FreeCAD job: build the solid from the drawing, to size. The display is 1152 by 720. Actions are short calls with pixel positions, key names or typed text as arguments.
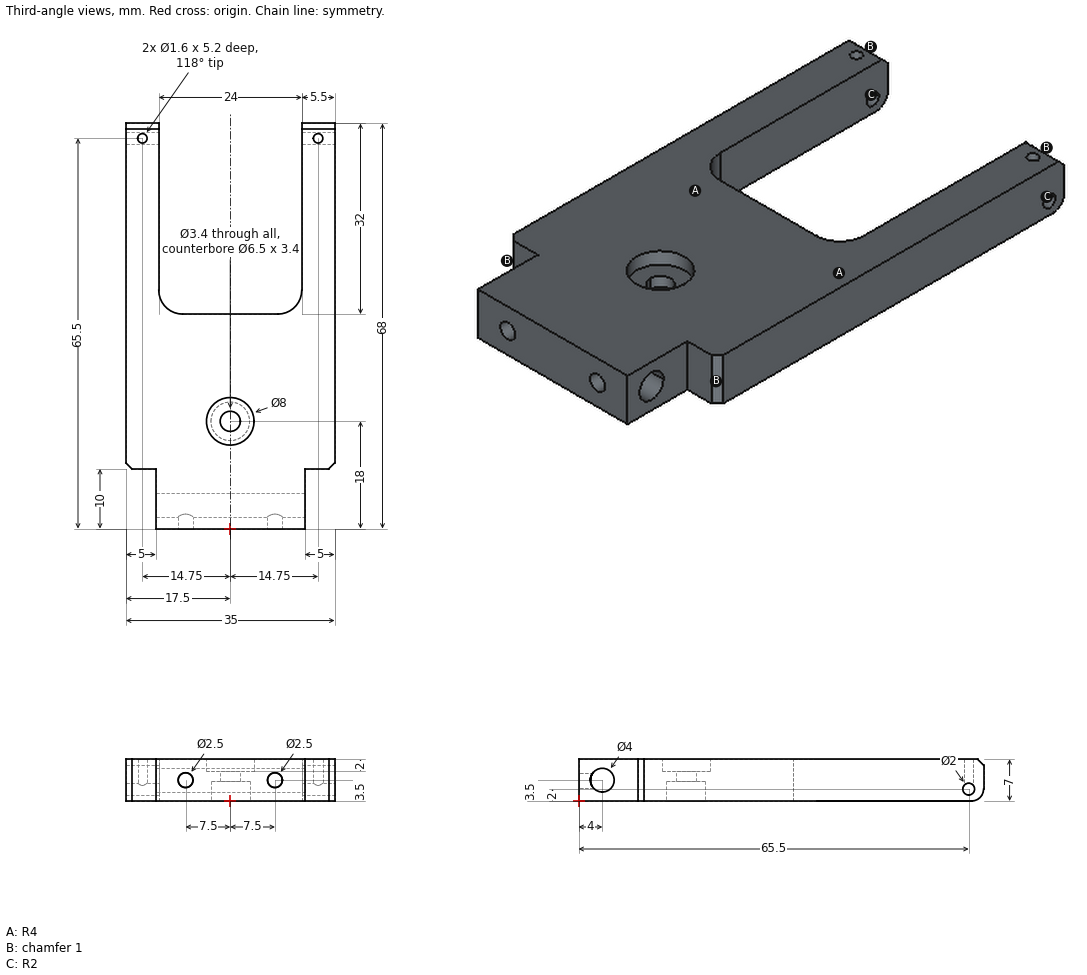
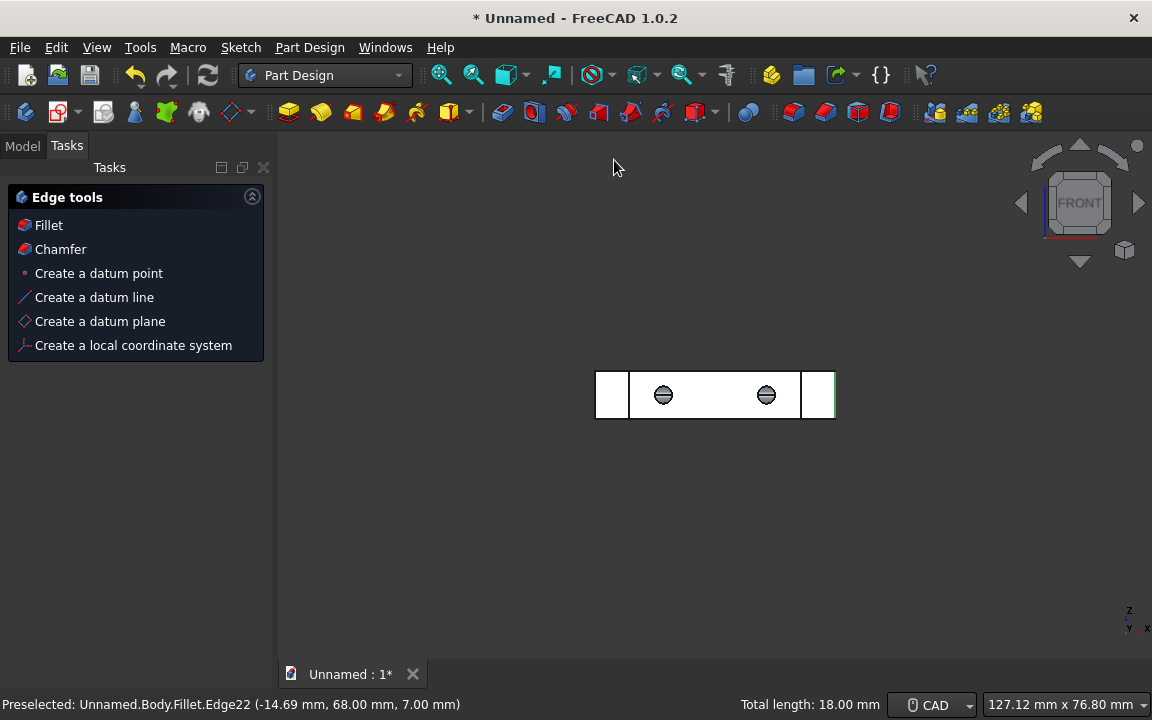
key(v)
key(f)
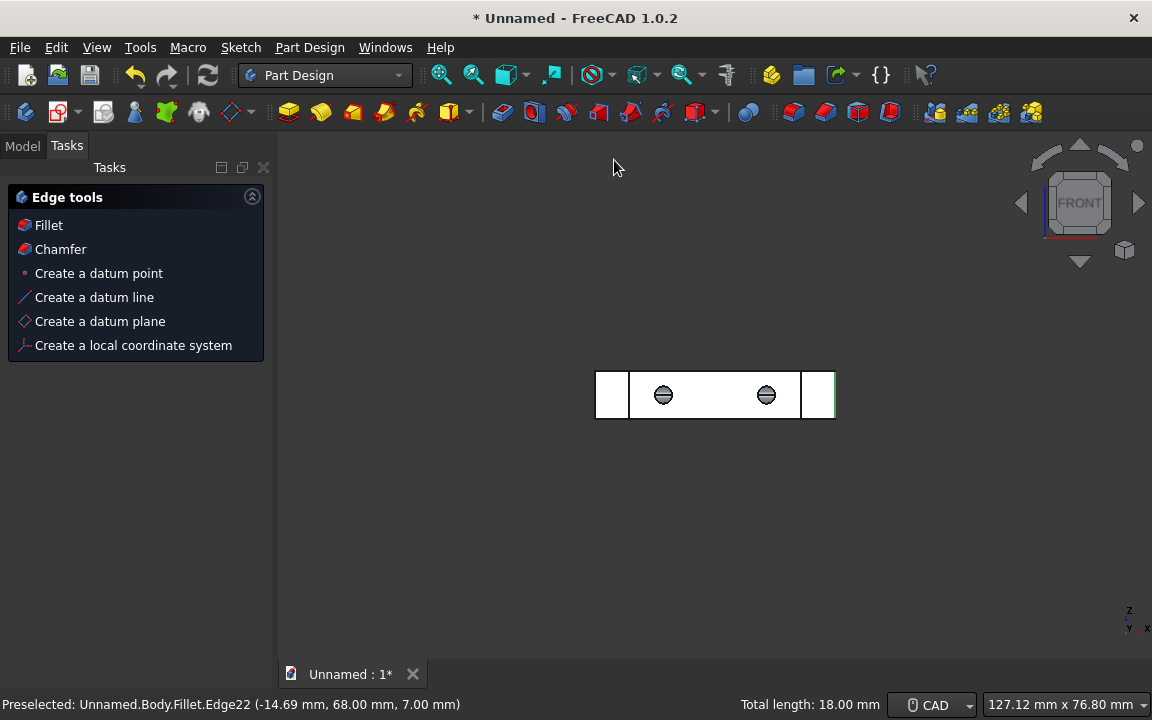
click(595, 394, ctrl)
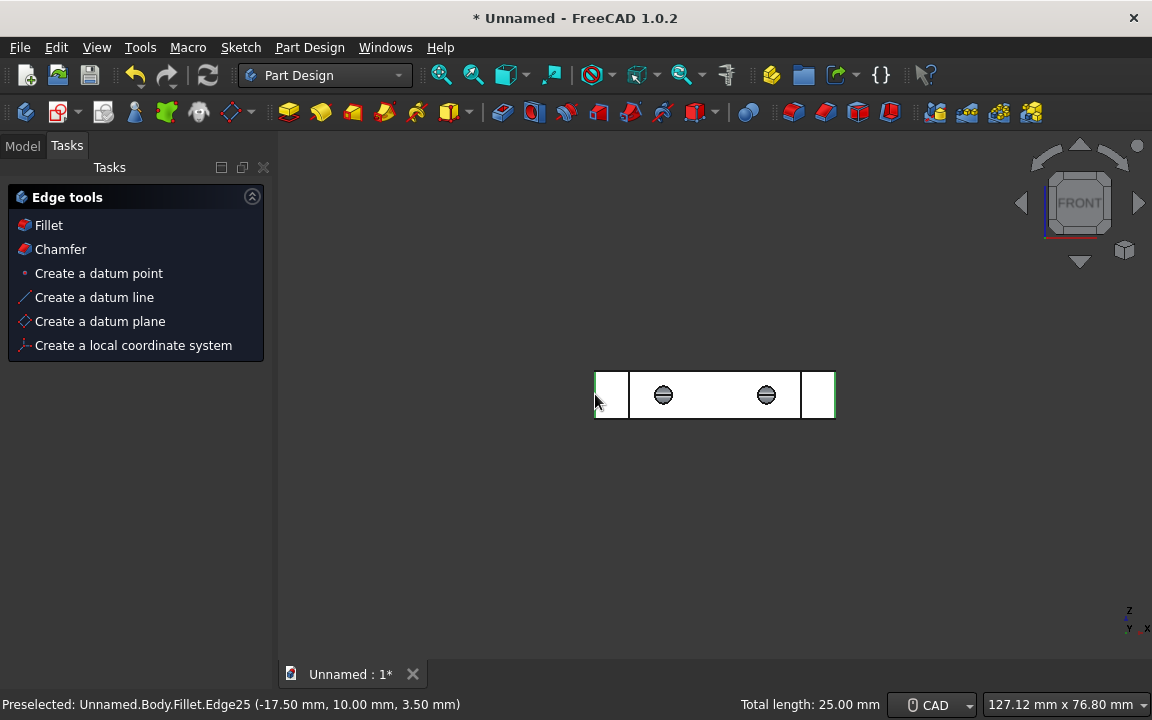
click(826, 112)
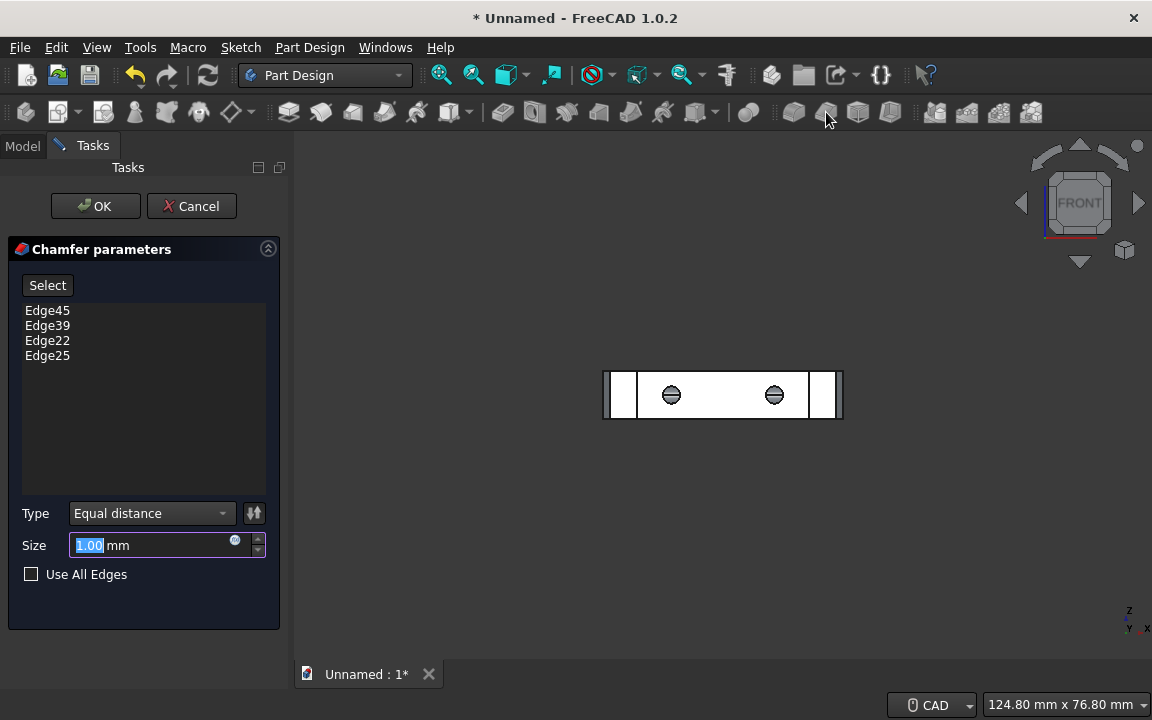
text(1)
key(Tab)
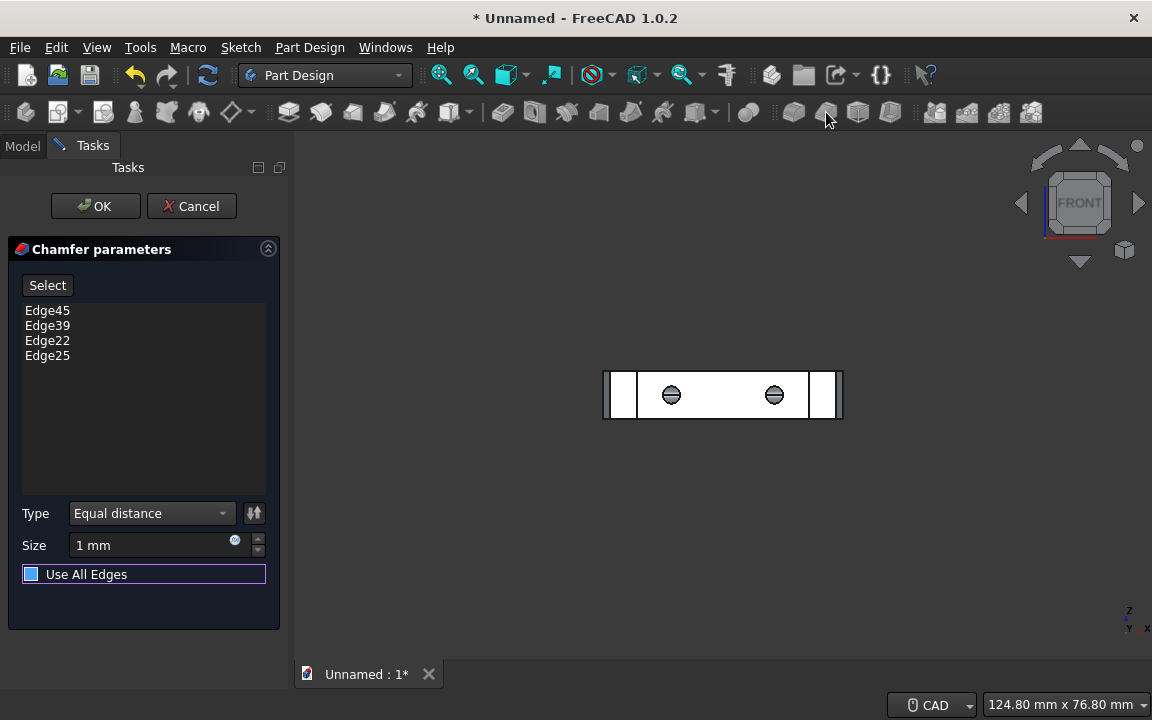
click(96, 206)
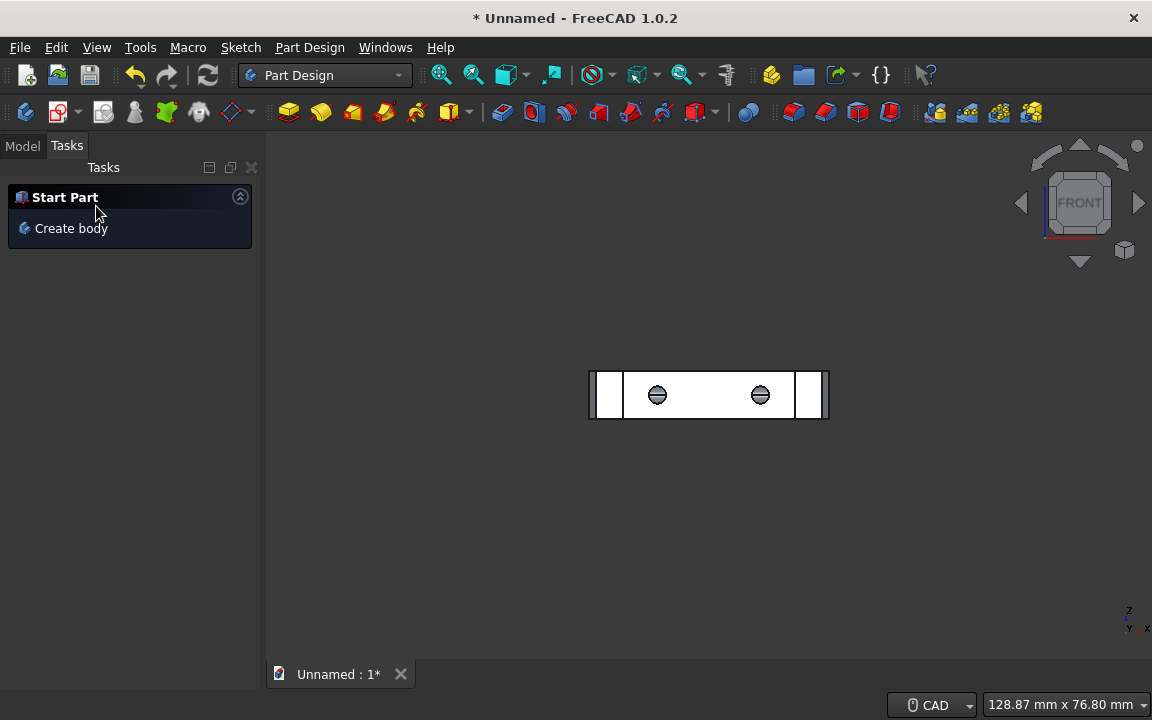
key(v)
key(f)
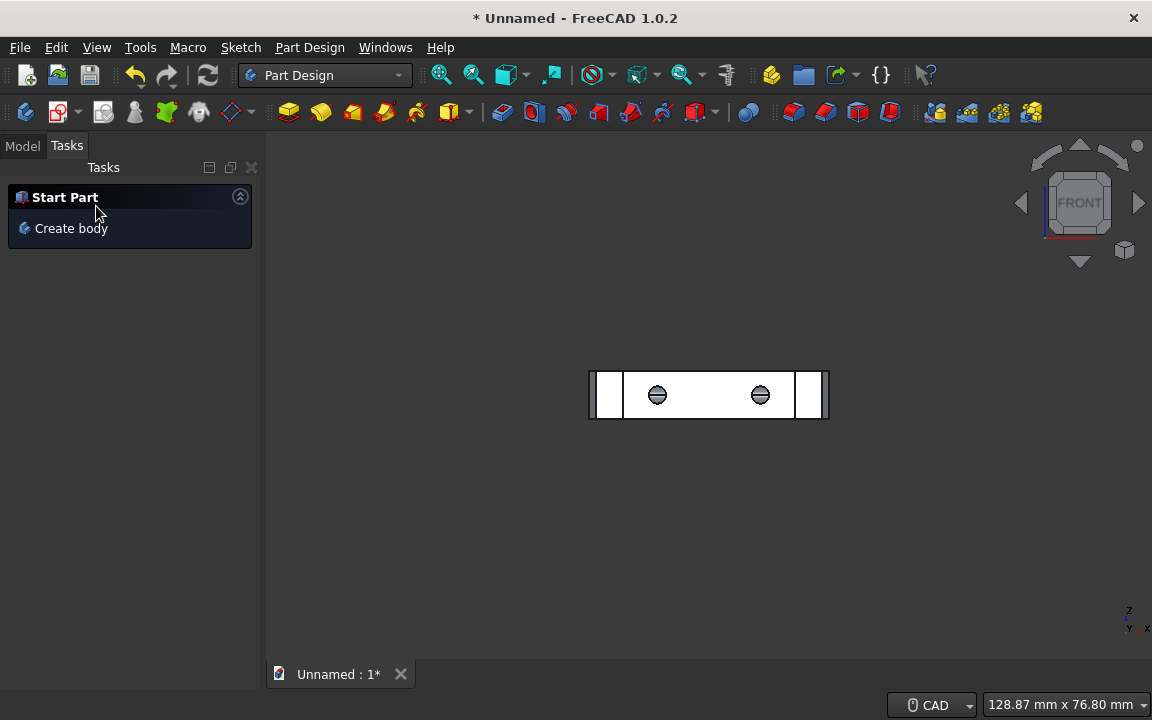
key(0)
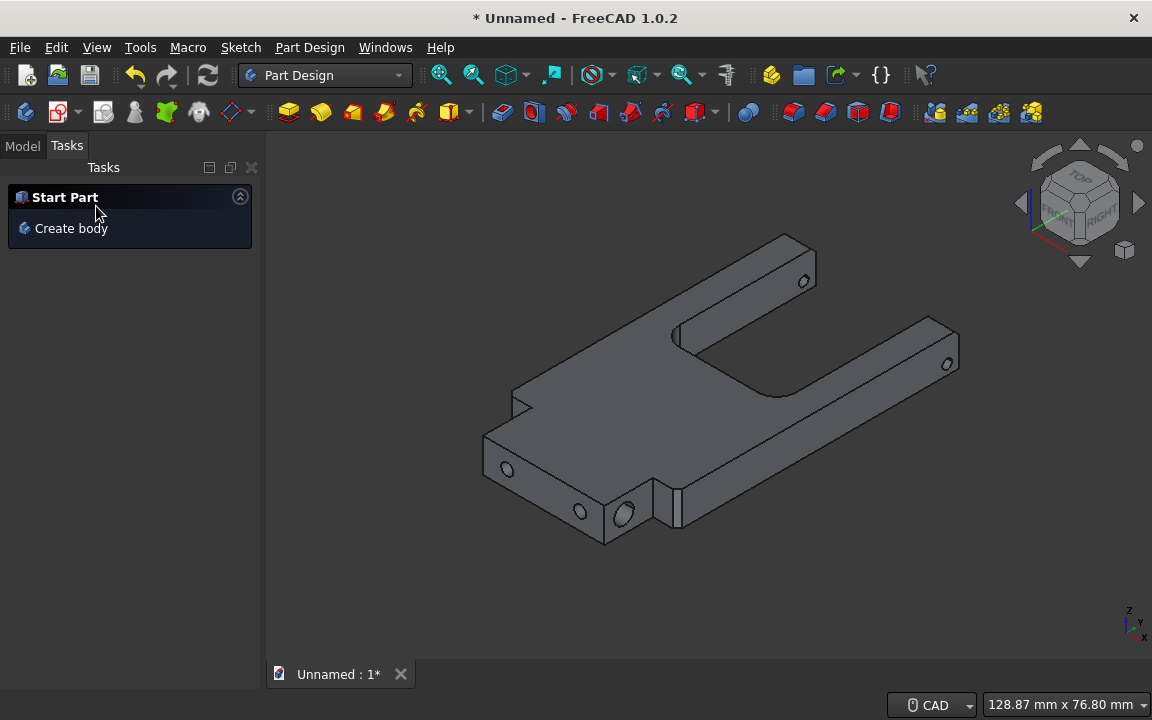
click(614, 429)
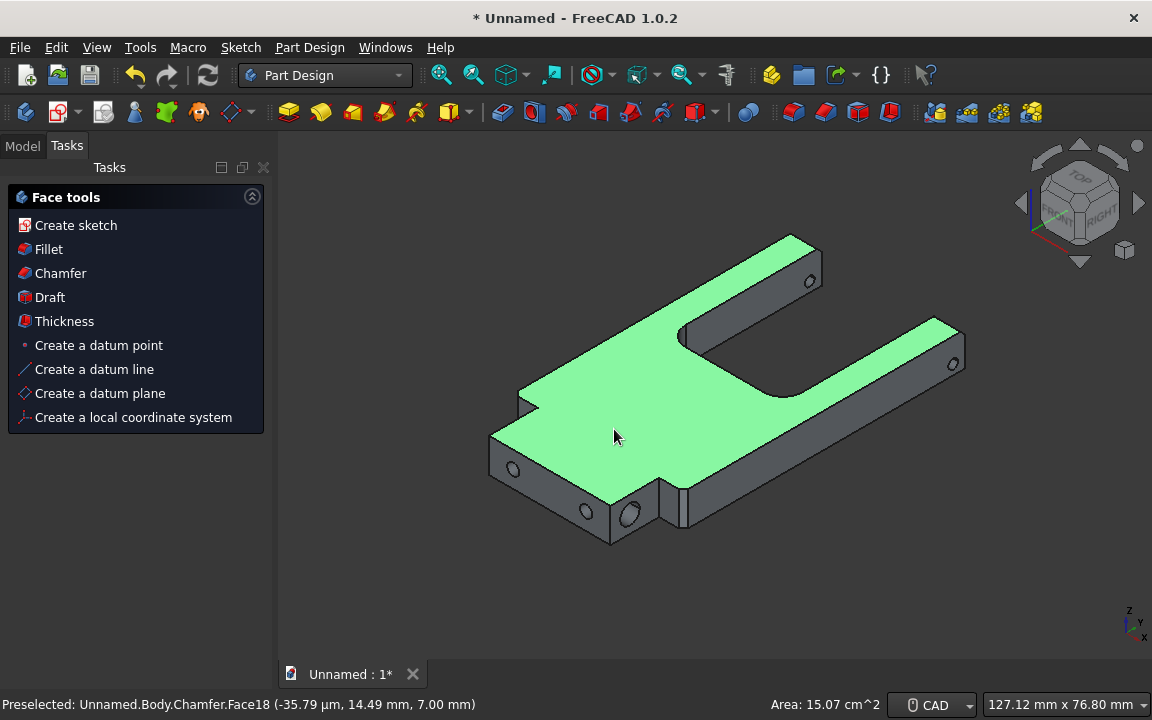
click(58, 112)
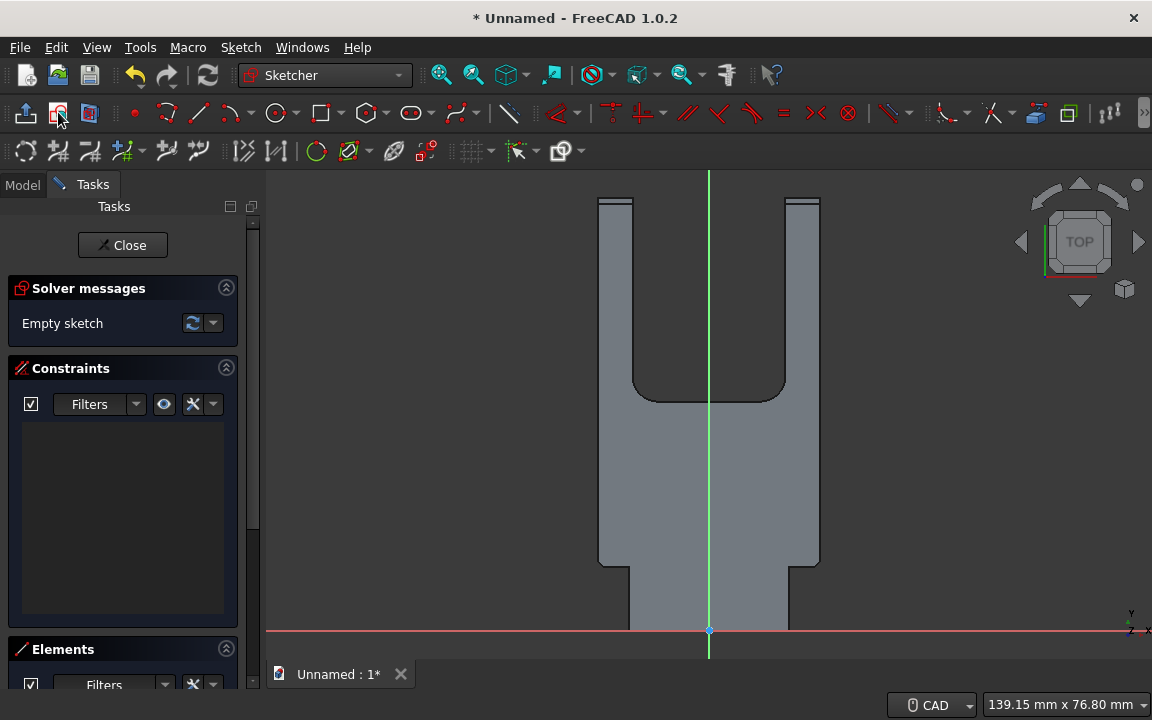
scroll(723, 537, up, 9)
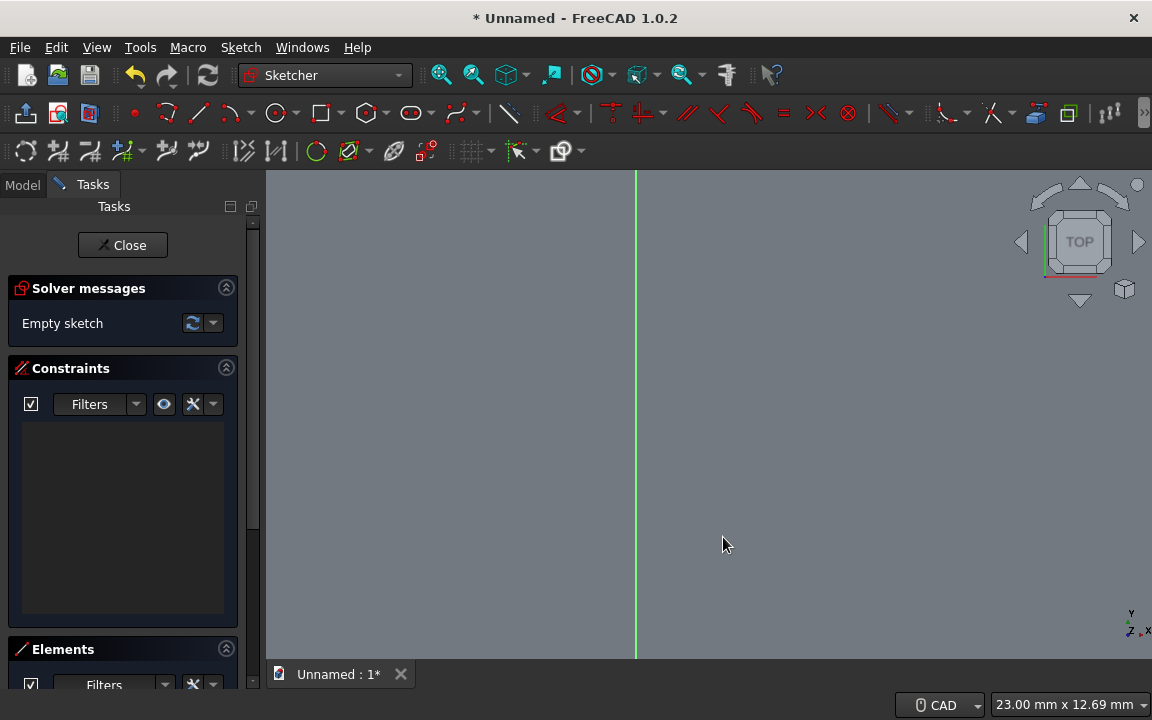
click(276, 114)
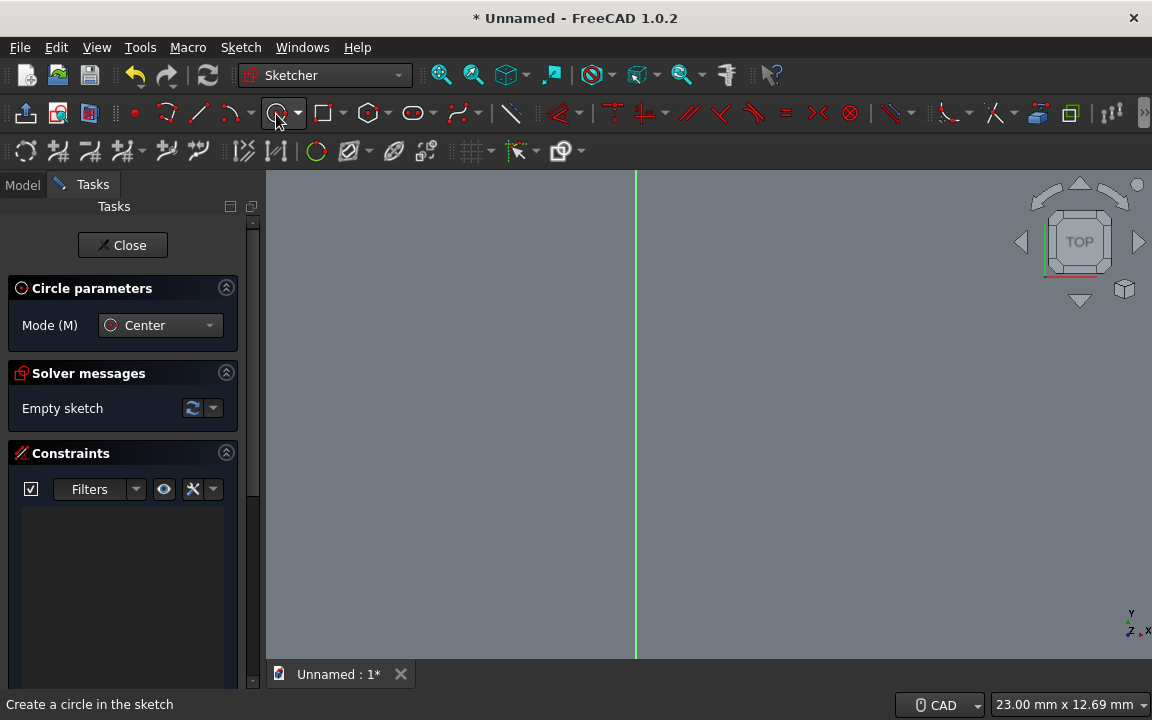
click(636, 408)
move(745, 299)